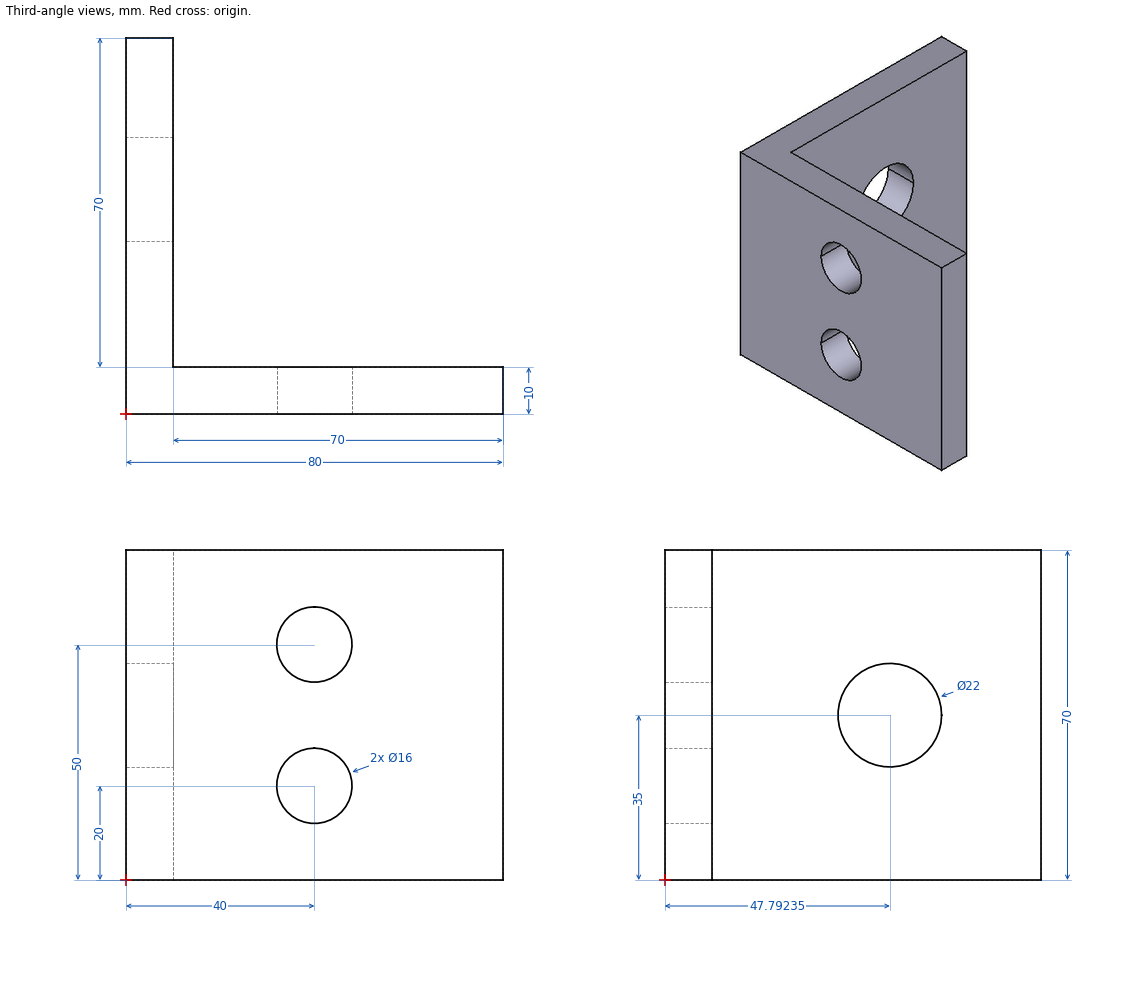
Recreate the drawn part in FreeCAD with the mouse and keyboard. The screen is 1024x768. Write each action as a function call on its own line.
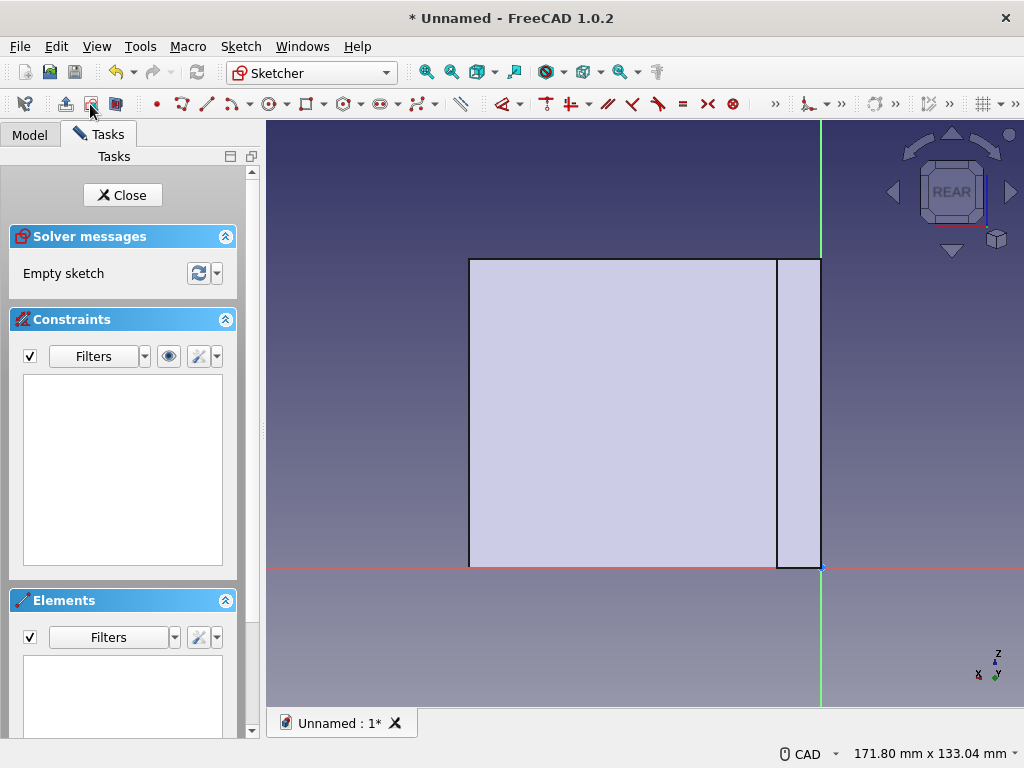
scroll(859, 494, up, 2)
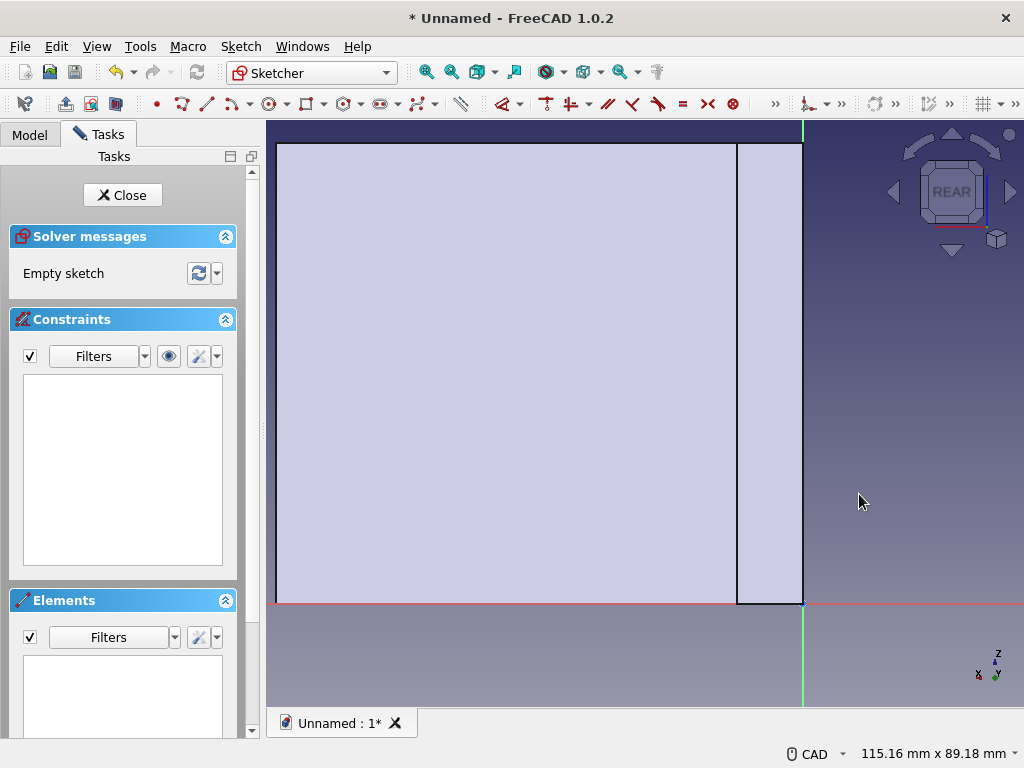
click(268, 104)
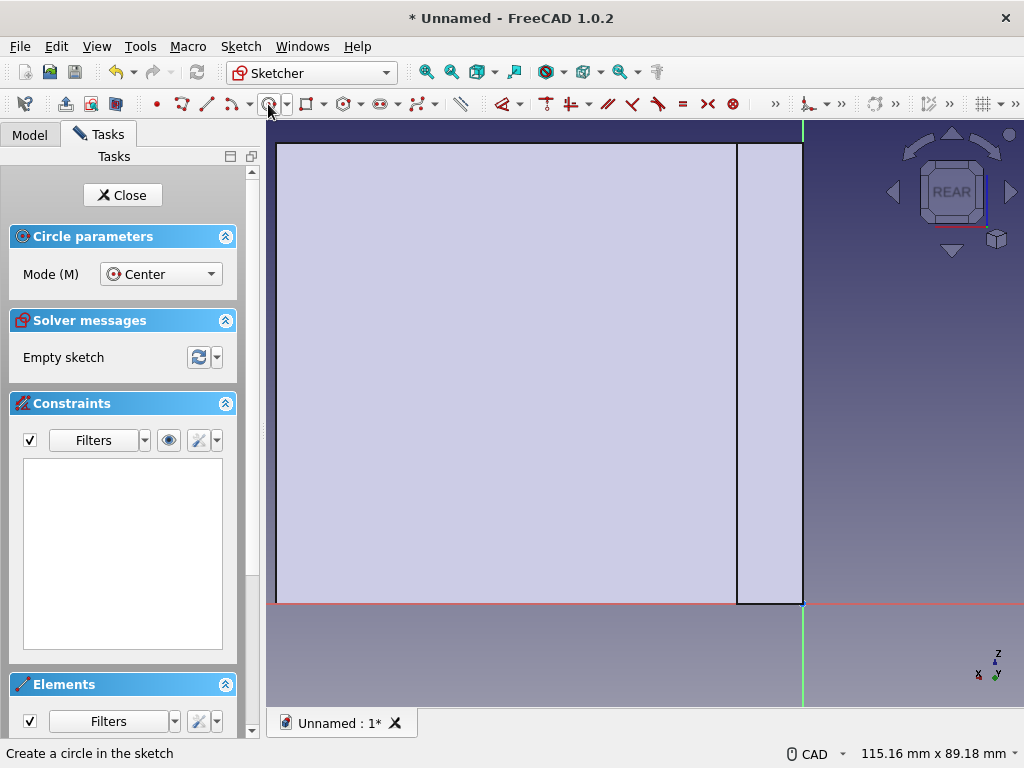
click(539, 472)
click(577, 435)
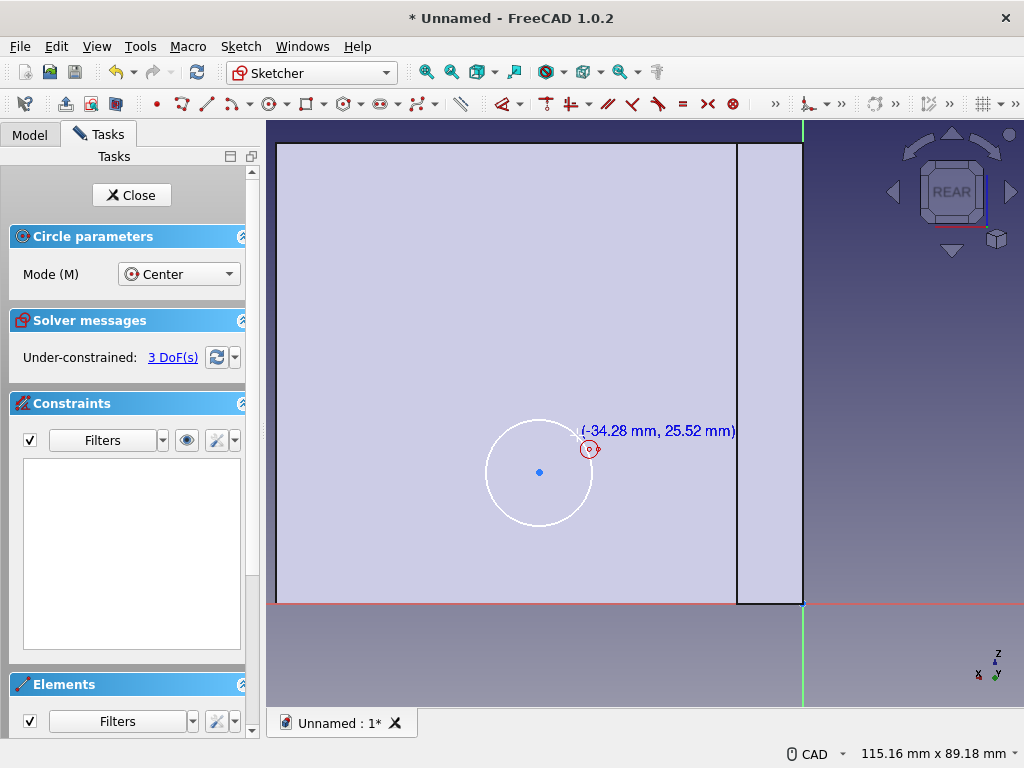
click(539, 275)
click(577, 238)
key(Escape)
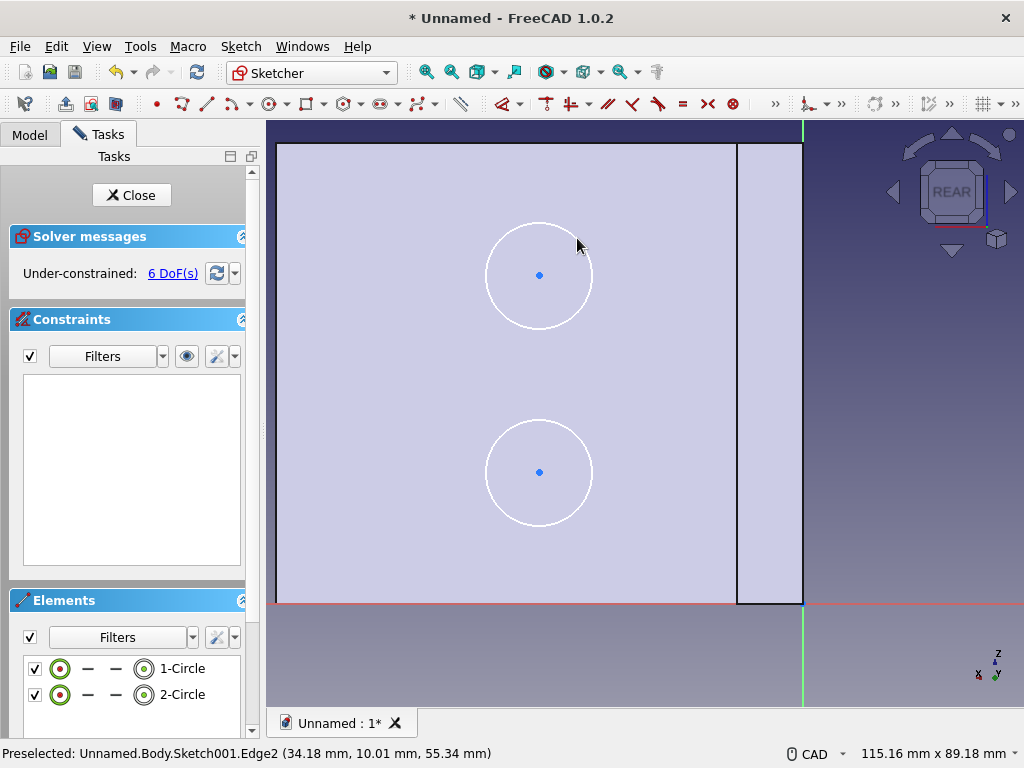
click(576, 435)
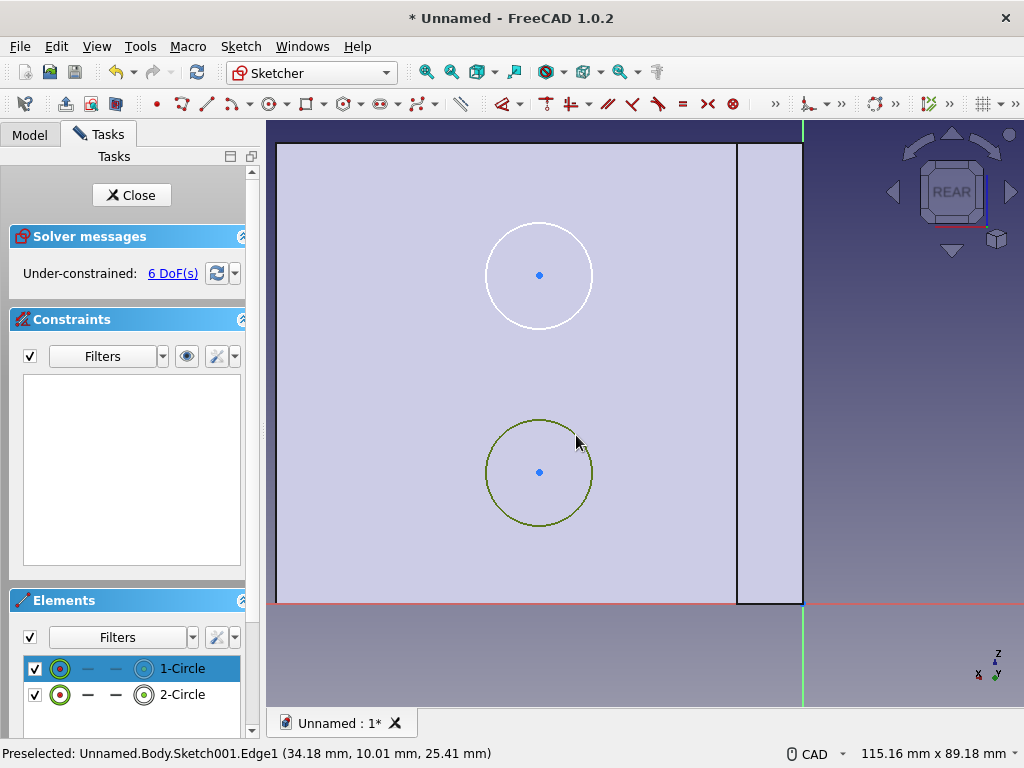
click(576, 238)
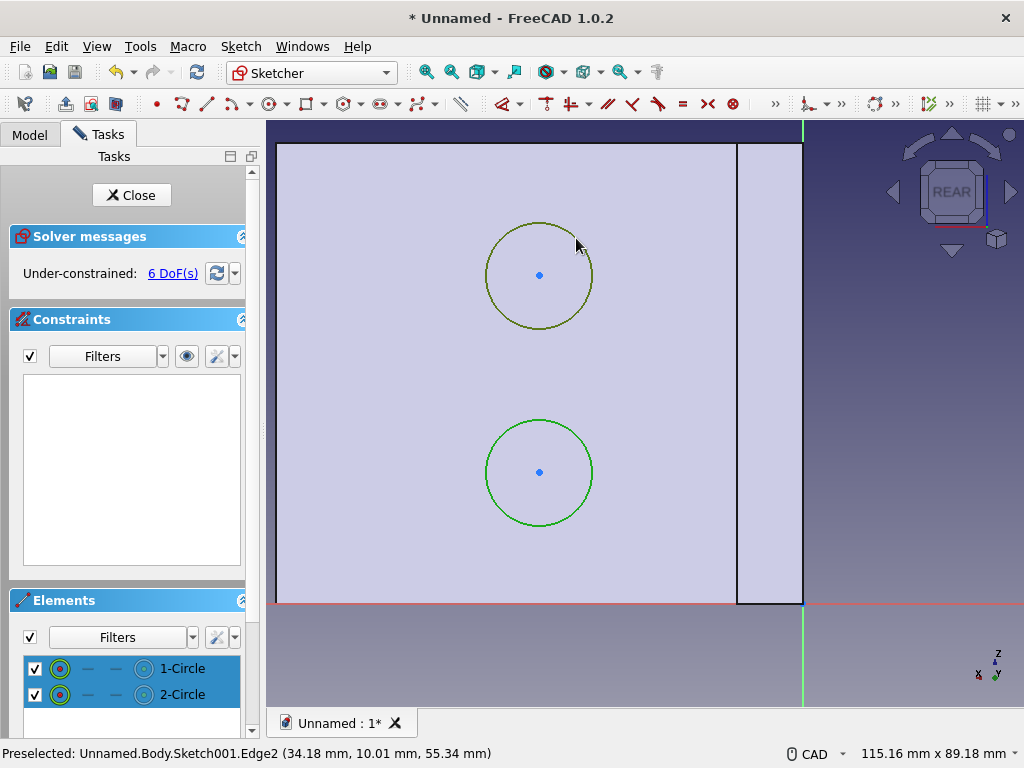
click(683, 104)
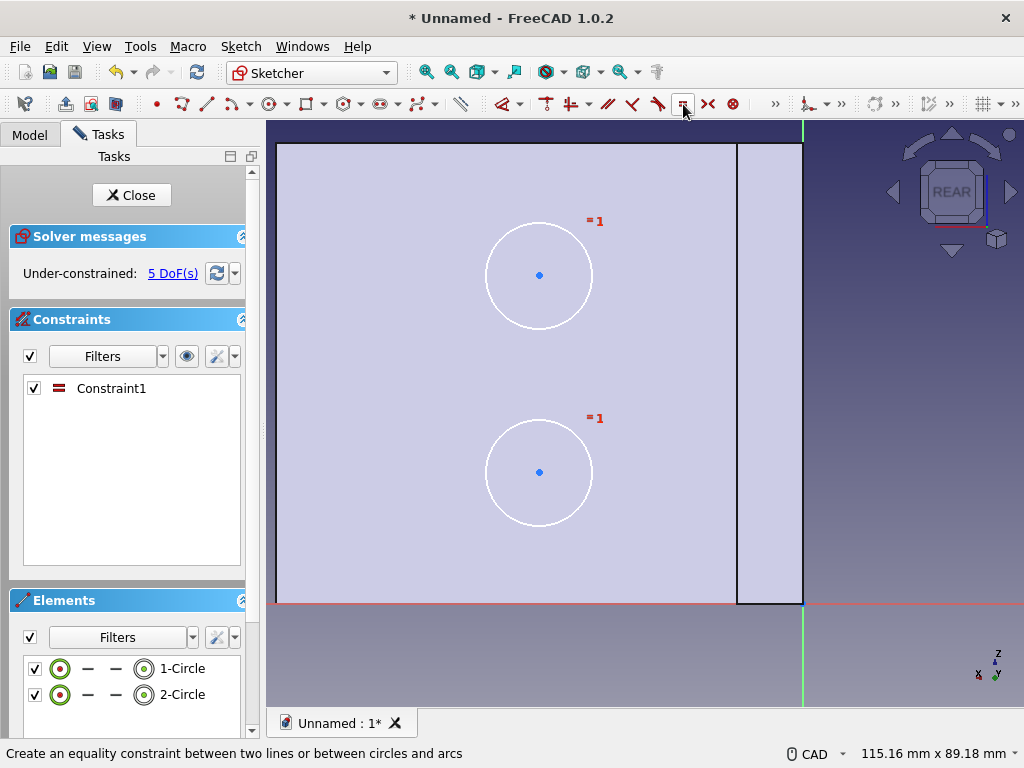
click(539, 473)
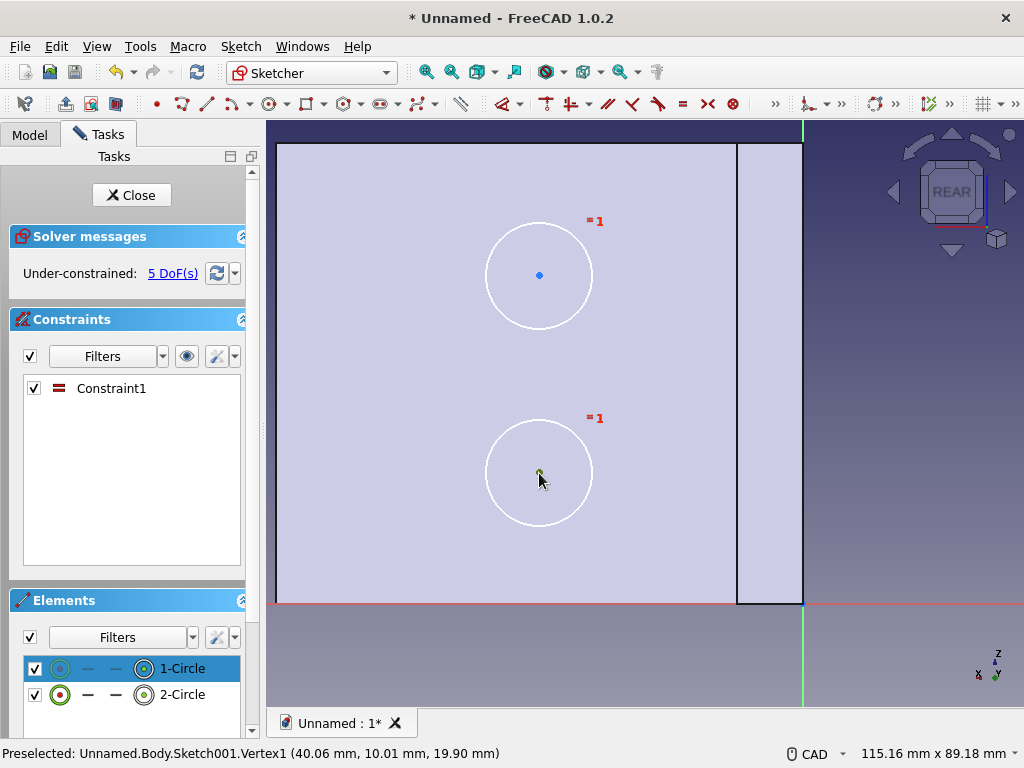
click(539, 276)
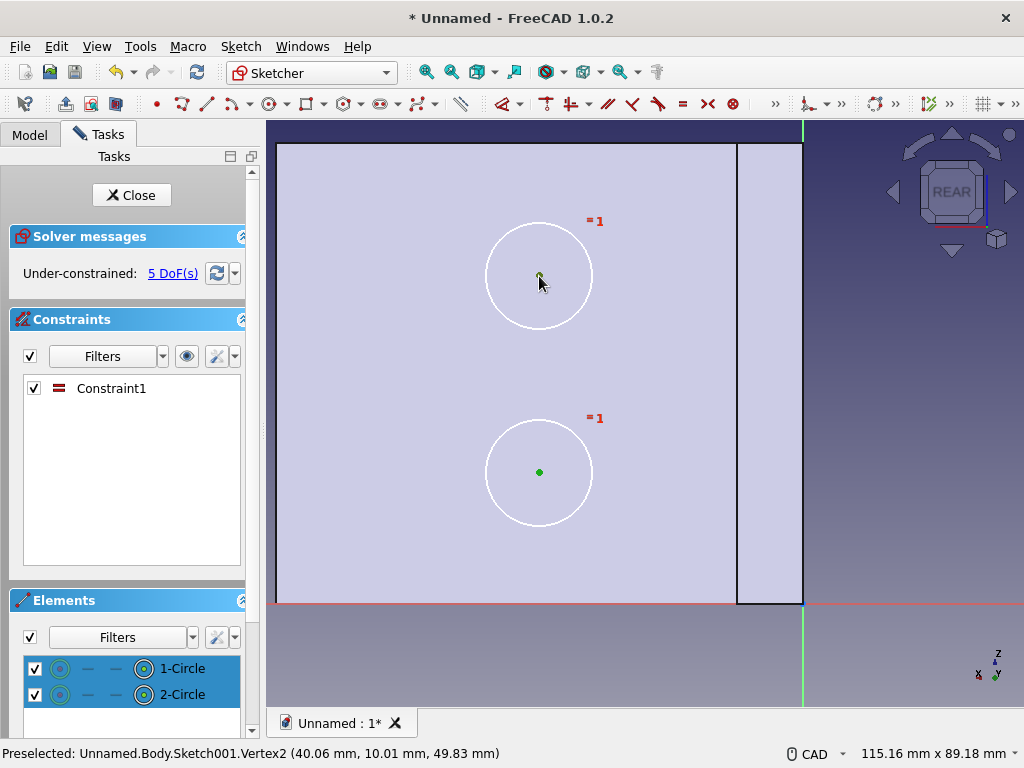
click(588, 104)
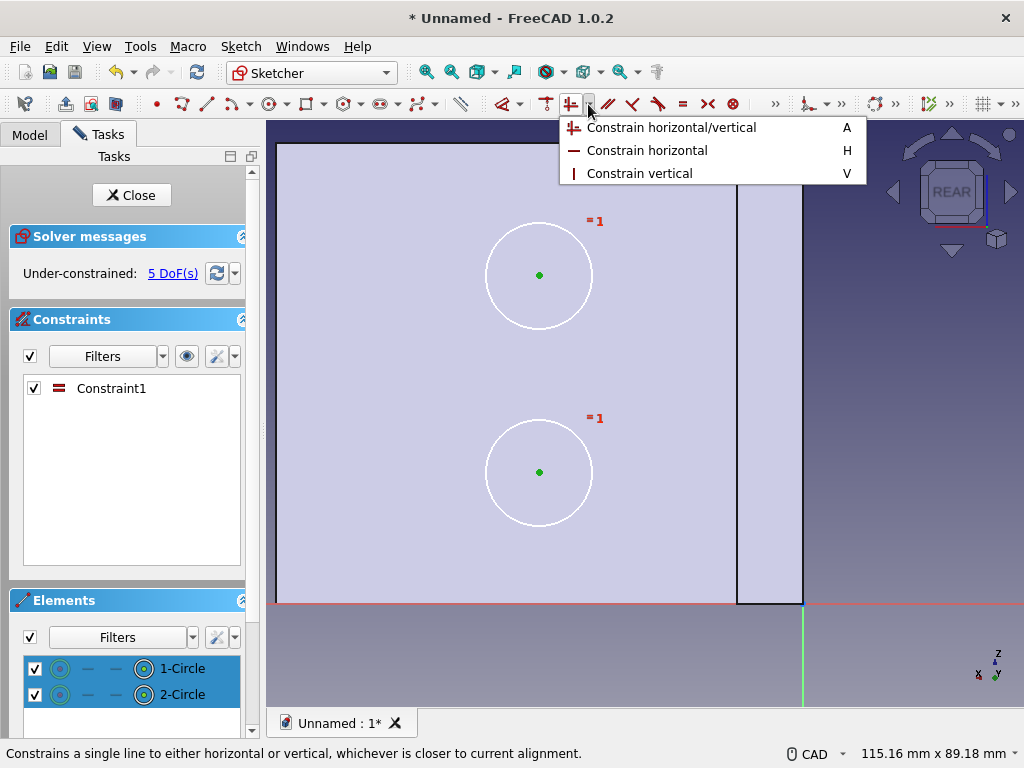
click(713, 174)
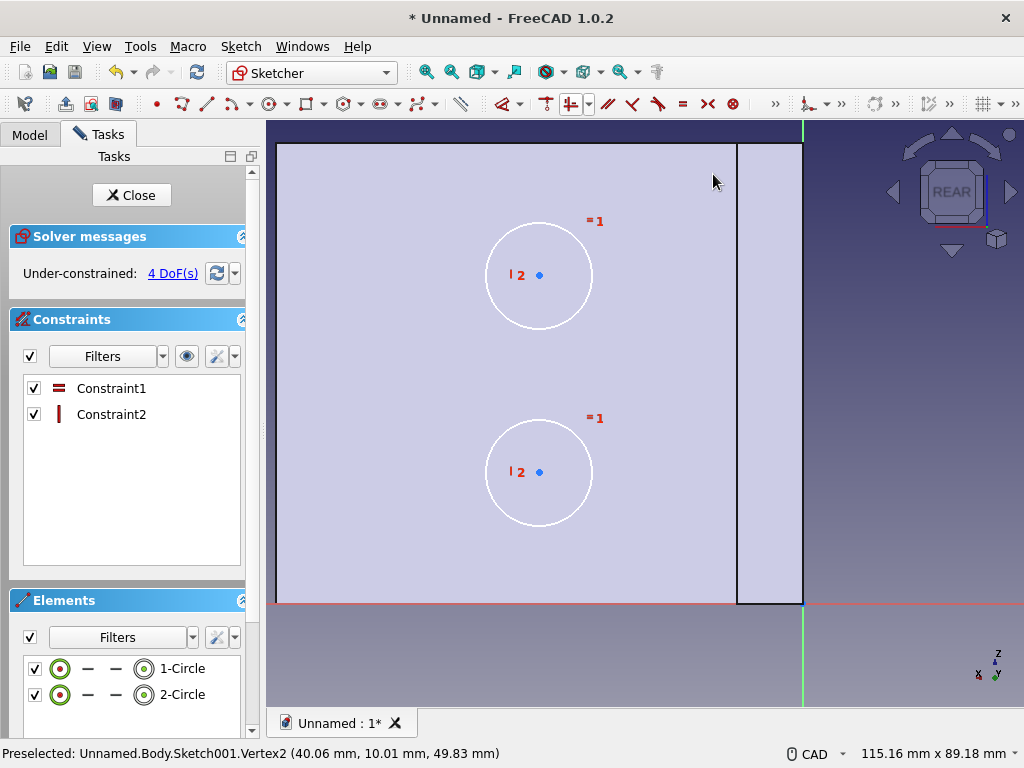
click(502, 104)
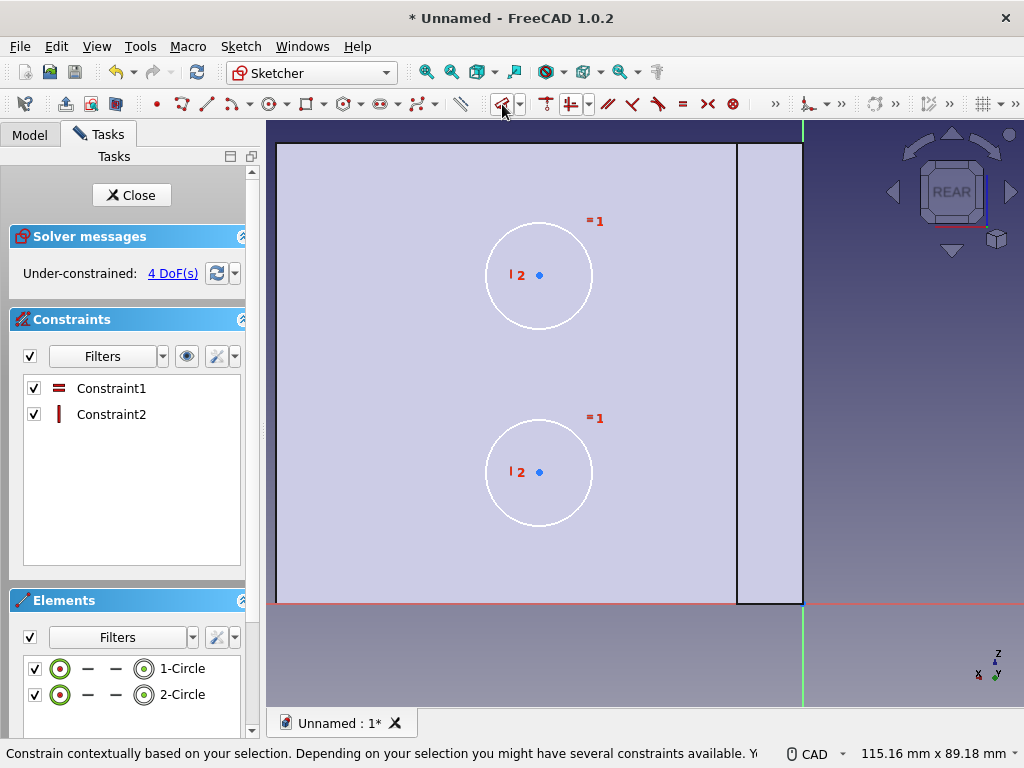
click(576, 435)
click(598, 412)